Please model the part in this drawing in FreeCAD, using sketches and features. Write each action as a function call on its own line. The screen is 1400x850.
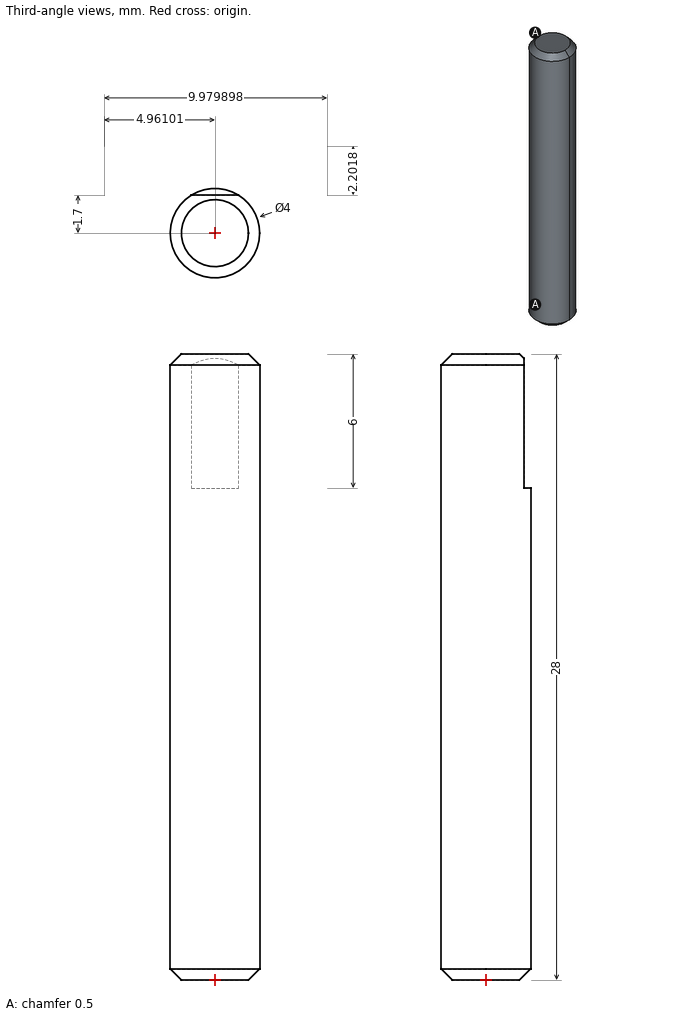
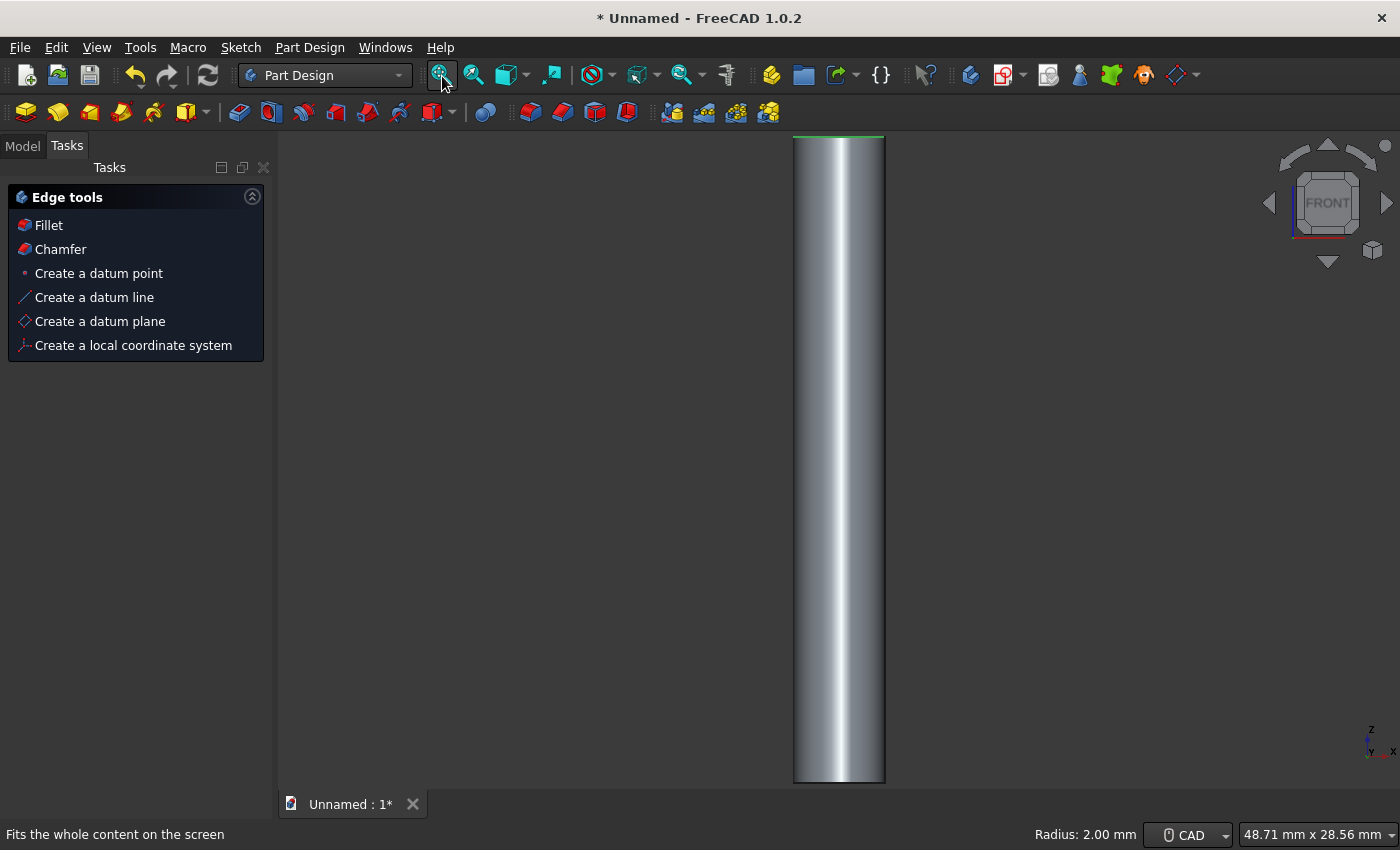
key(3)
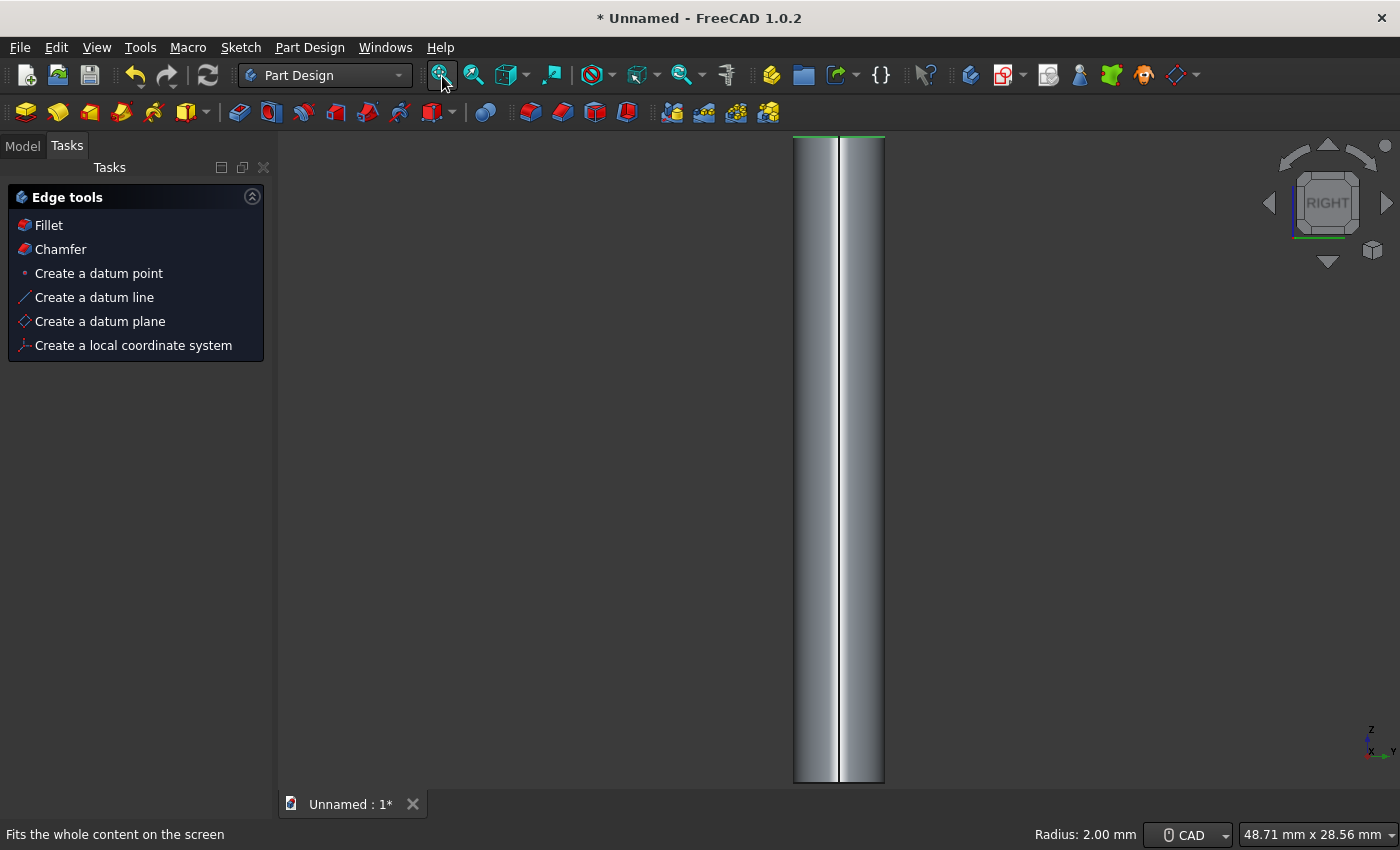
key(5)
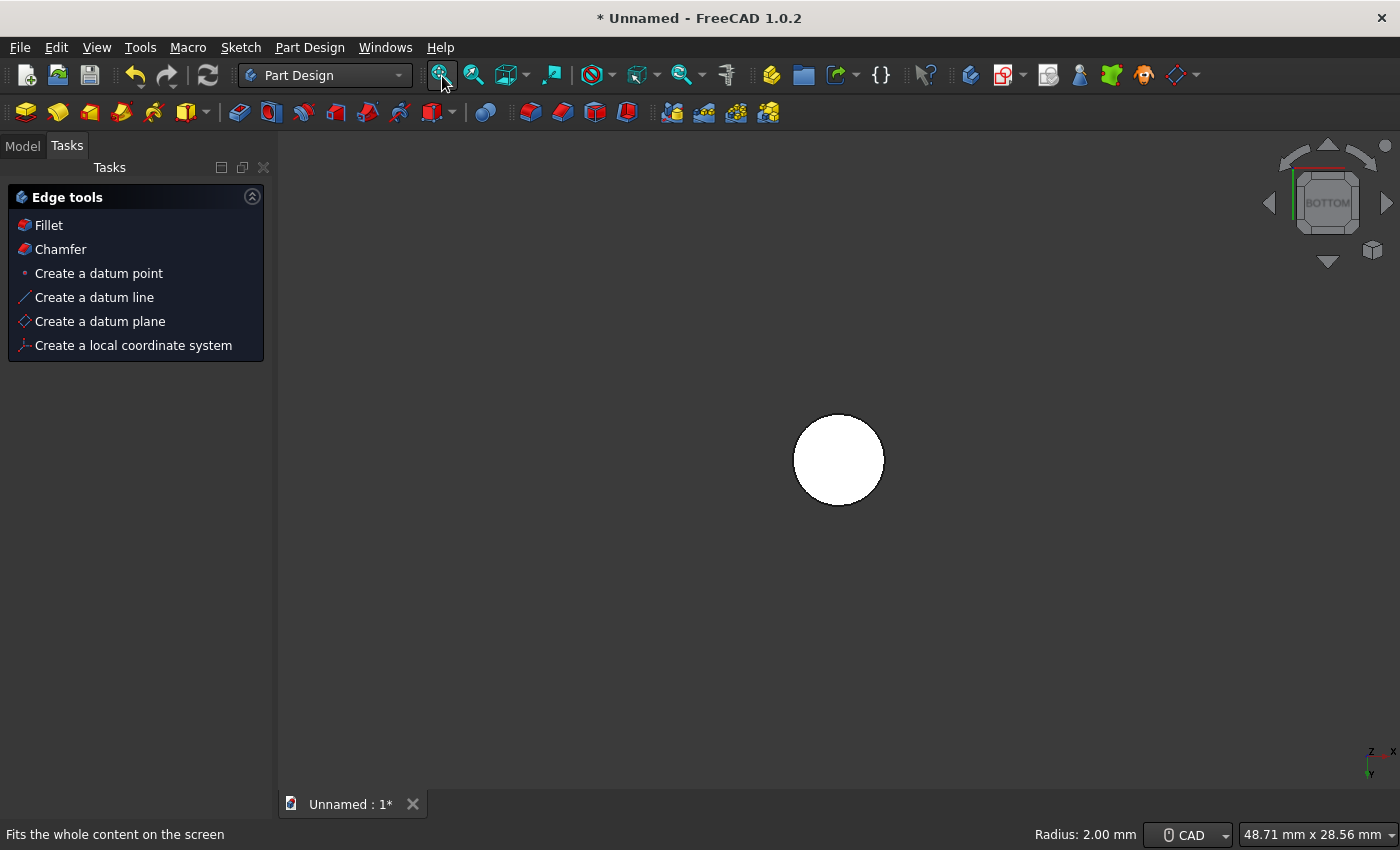
click(442, 76)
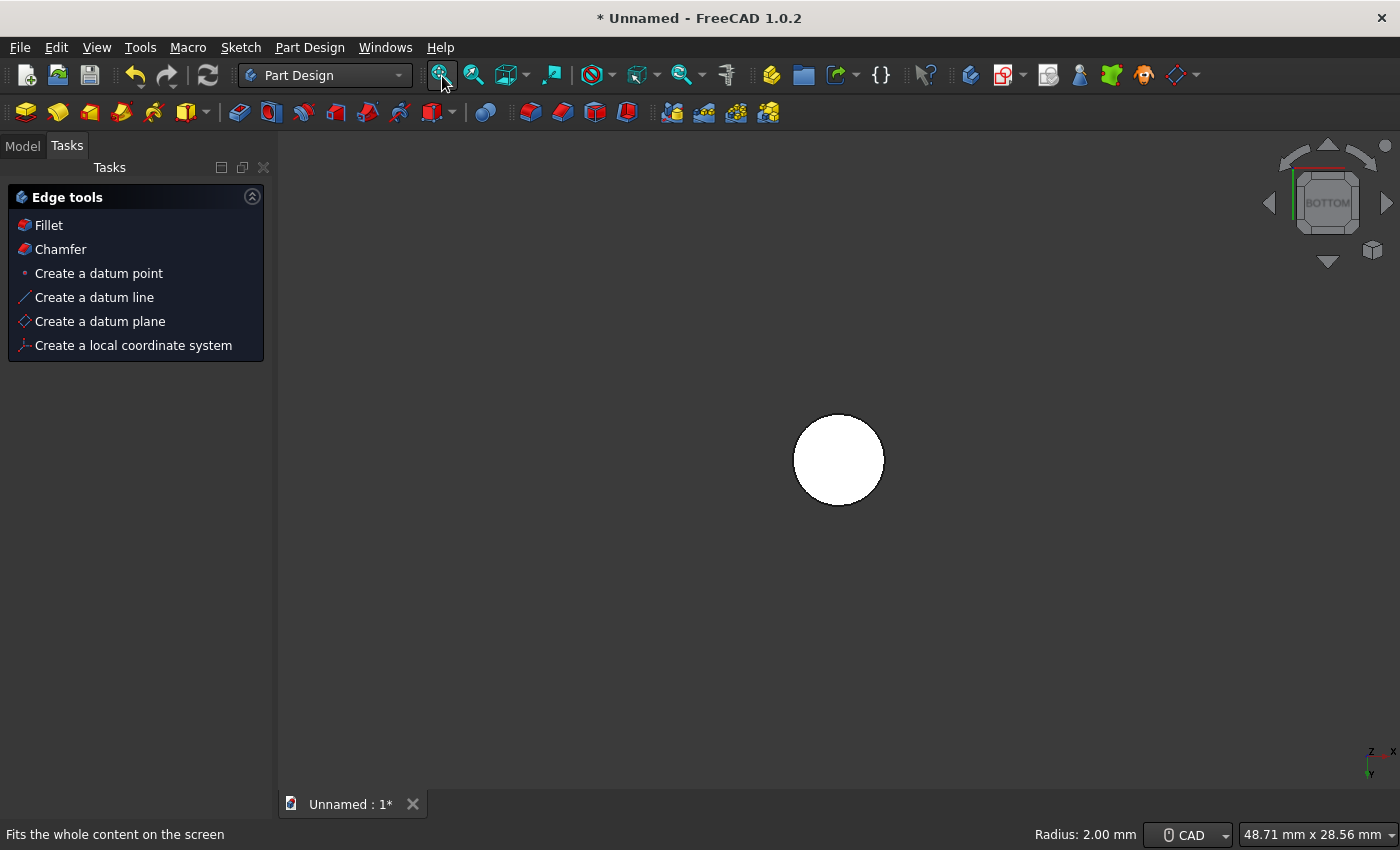
click(793, 459, ctrl)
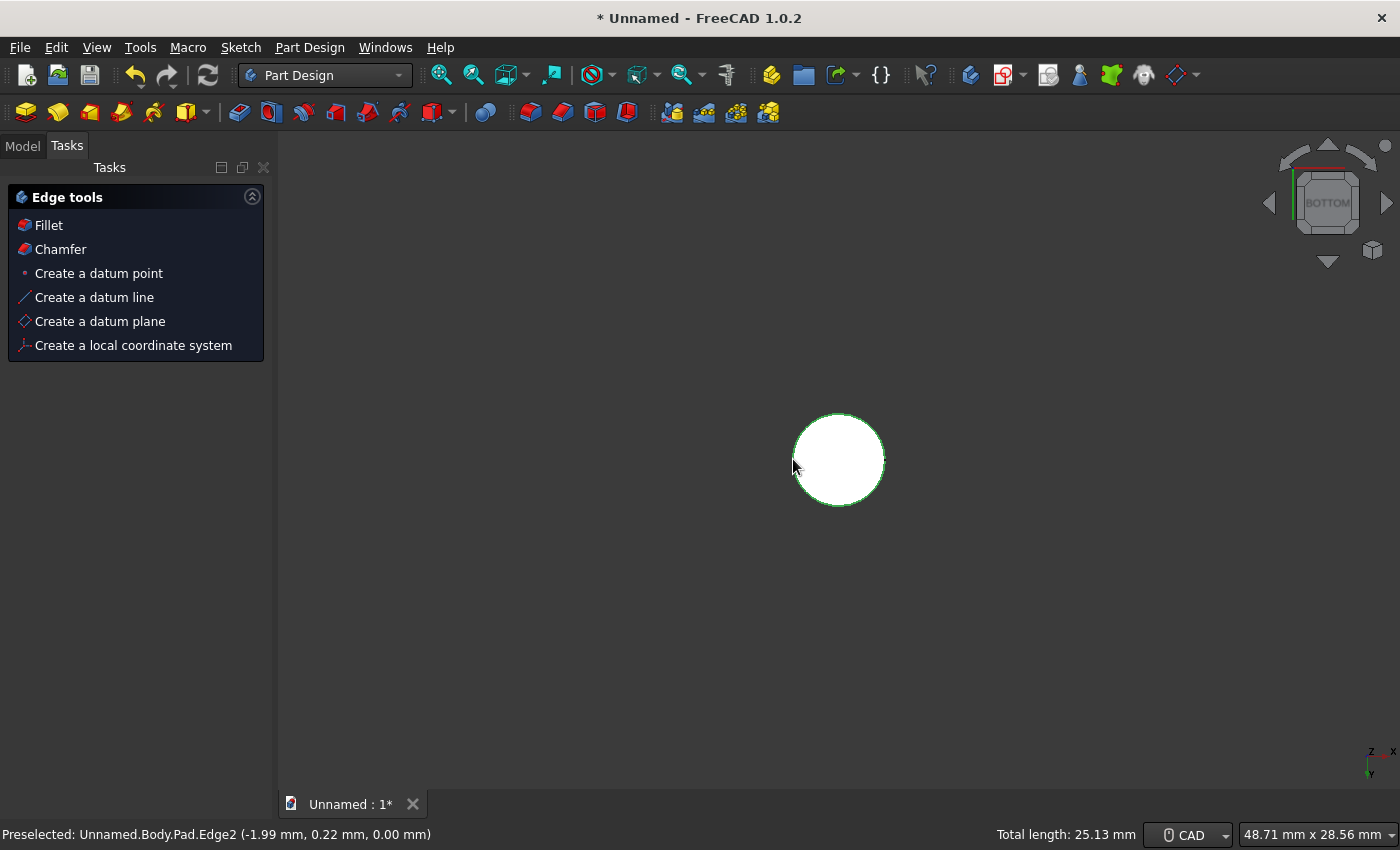
click(564, 112)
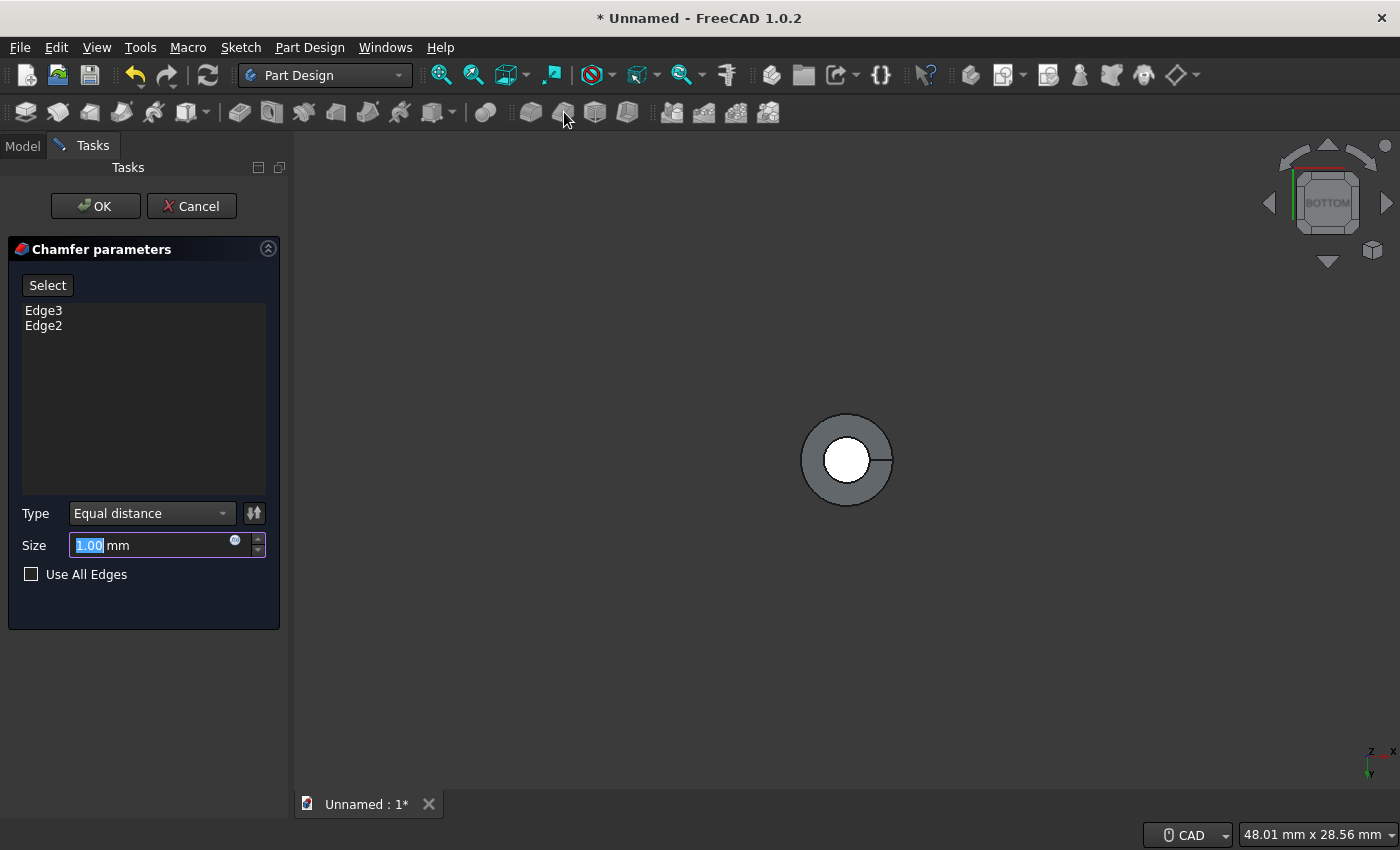
text(0.5)
key(Tab)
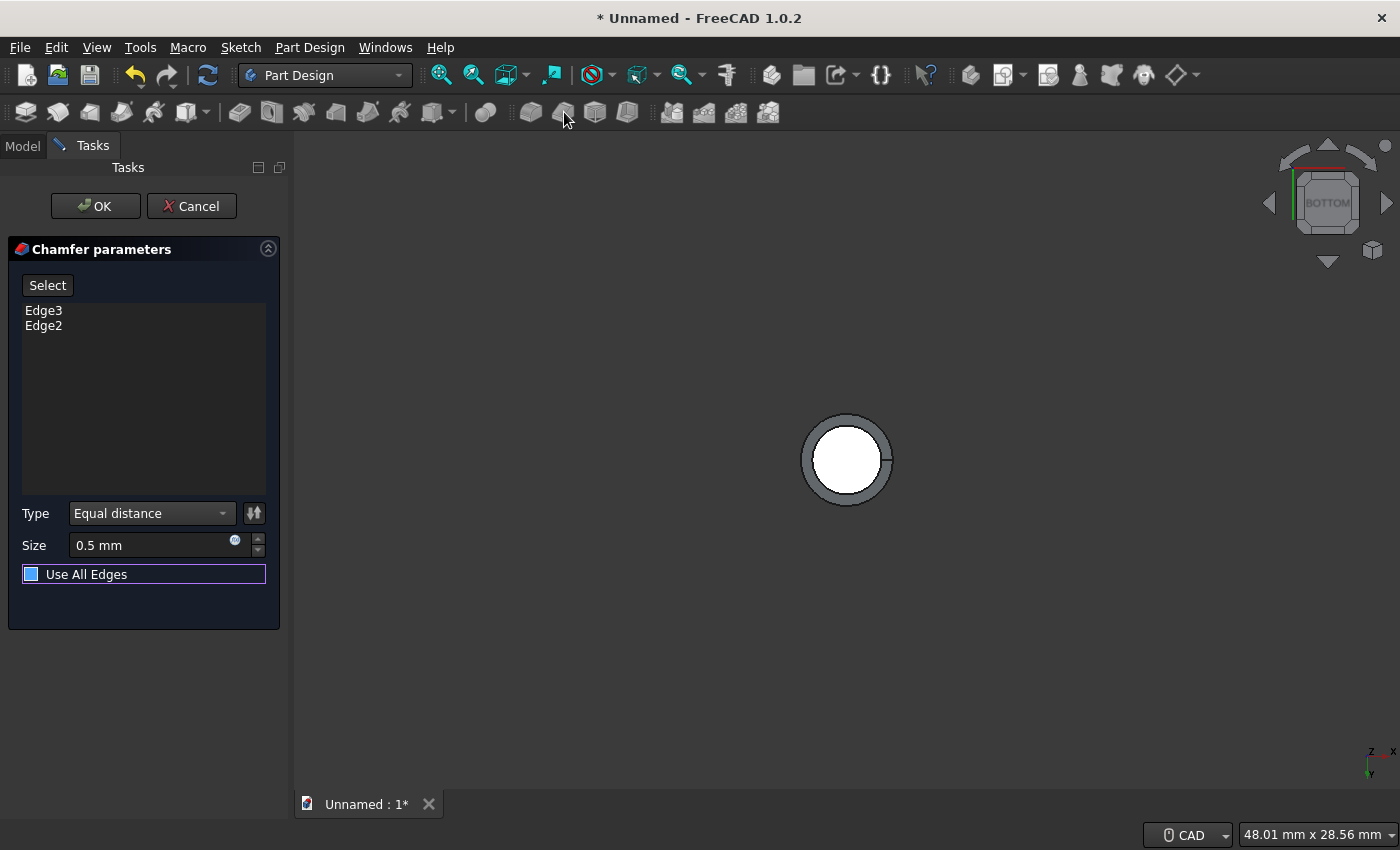
click(96, 206)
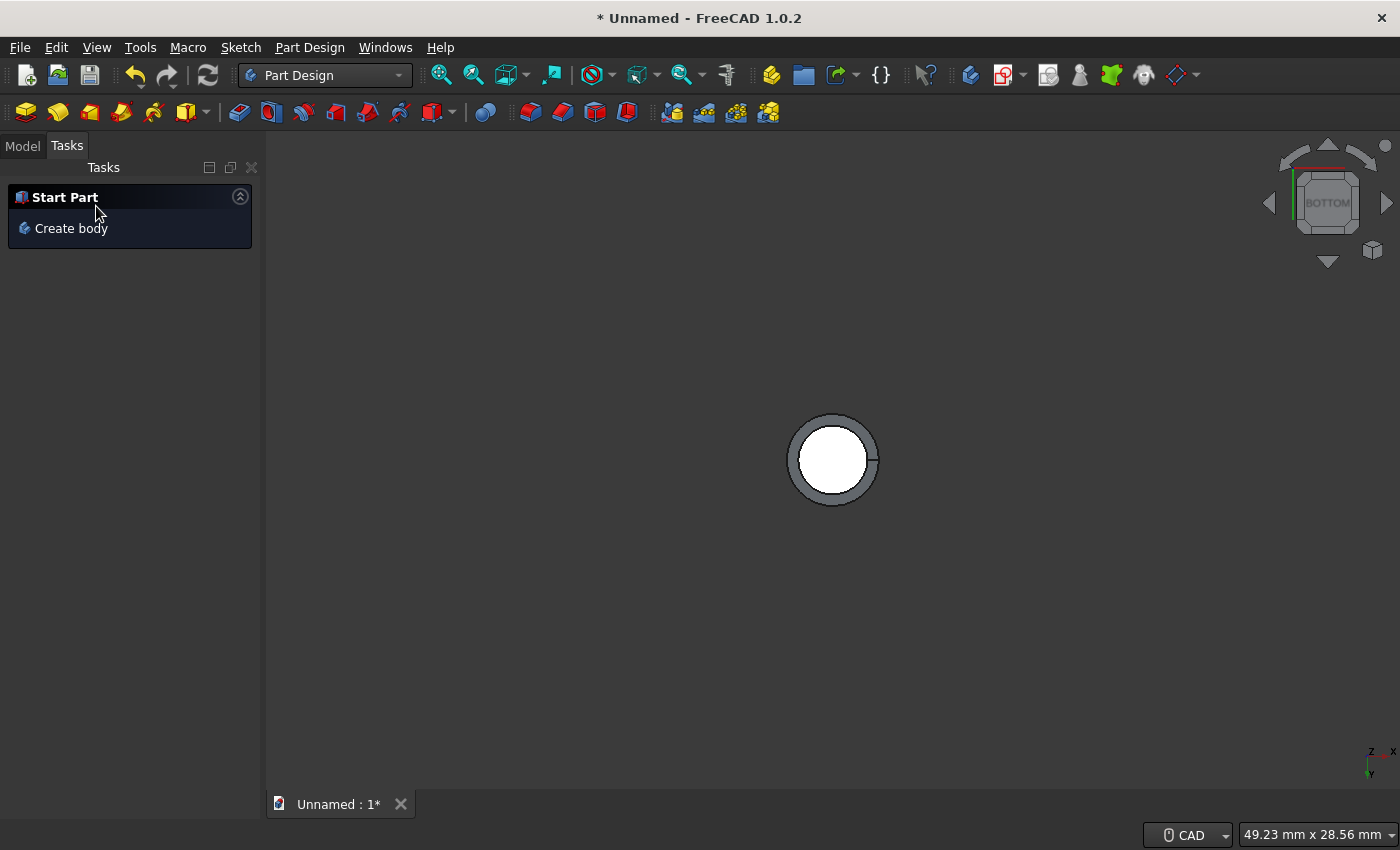
click(442, 76)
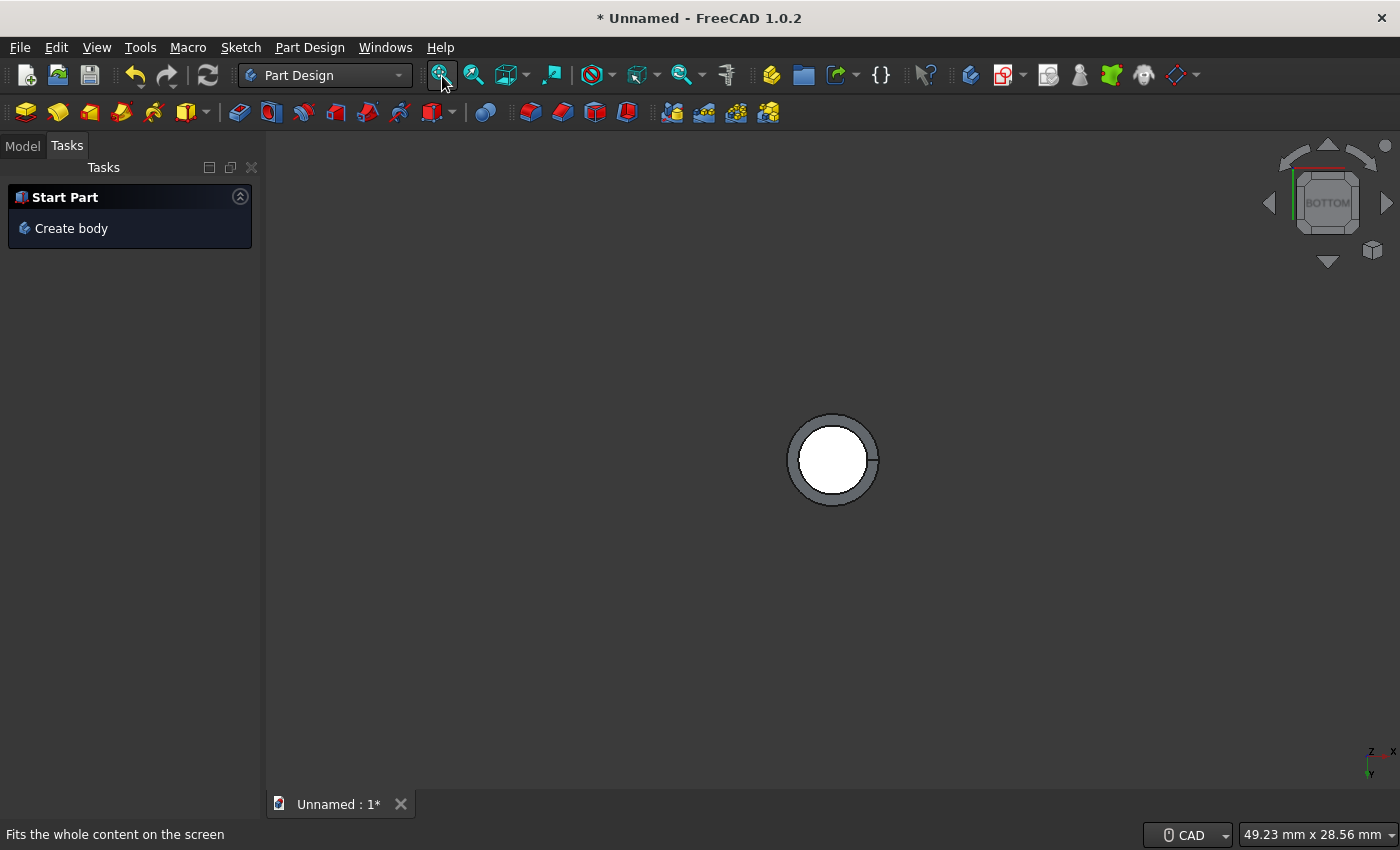
key(0)